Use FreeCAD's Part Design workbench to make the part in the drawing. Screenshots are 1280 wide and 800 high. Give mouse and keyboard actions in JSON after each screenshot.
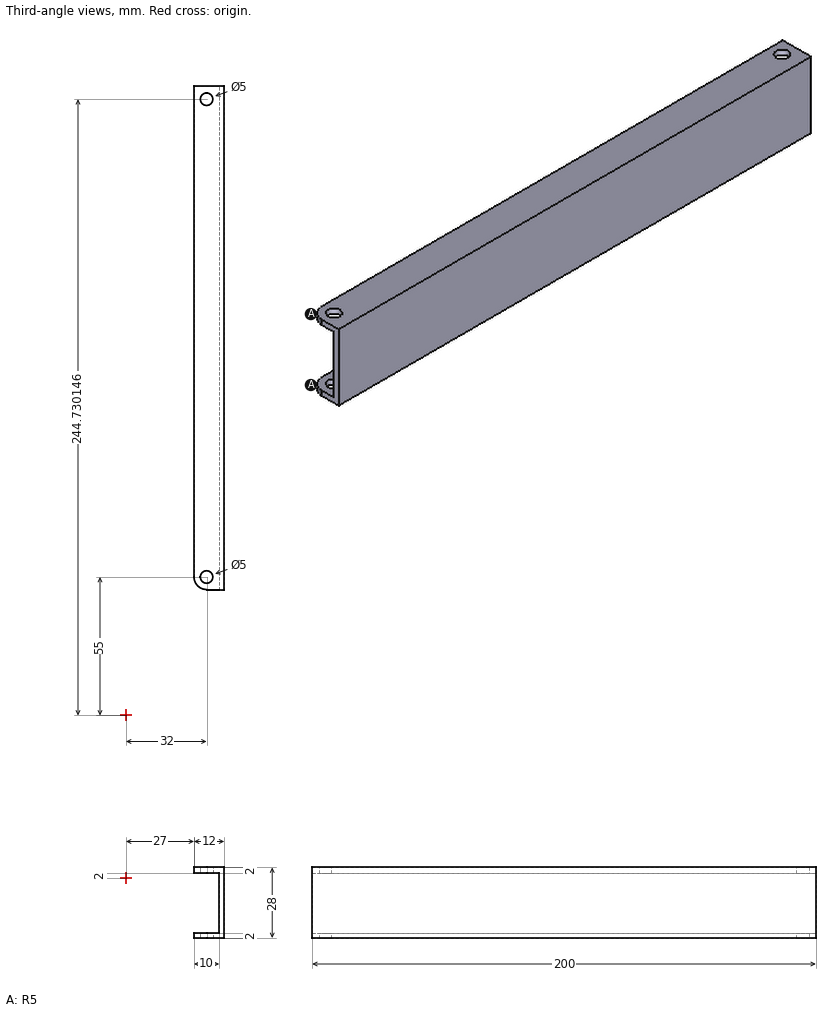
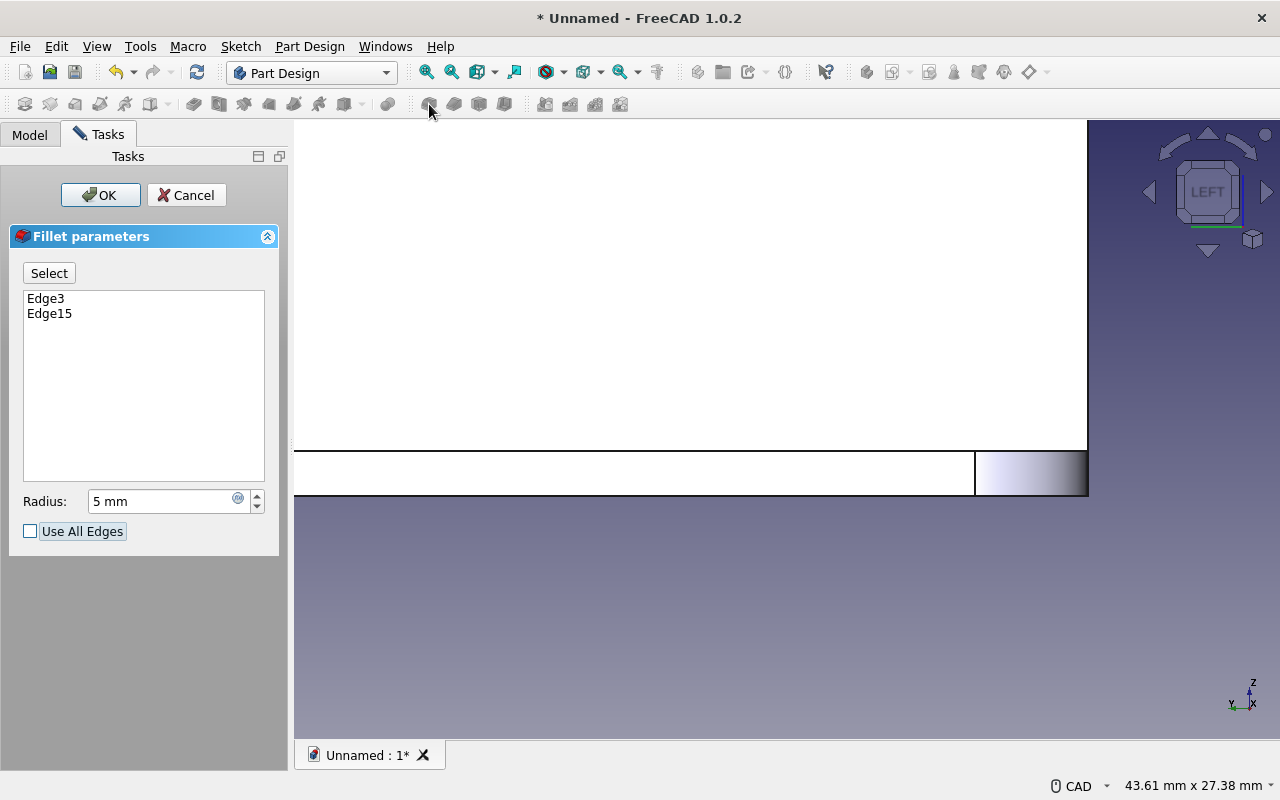
{"action": "left_click", "coordinate": [101, 195]}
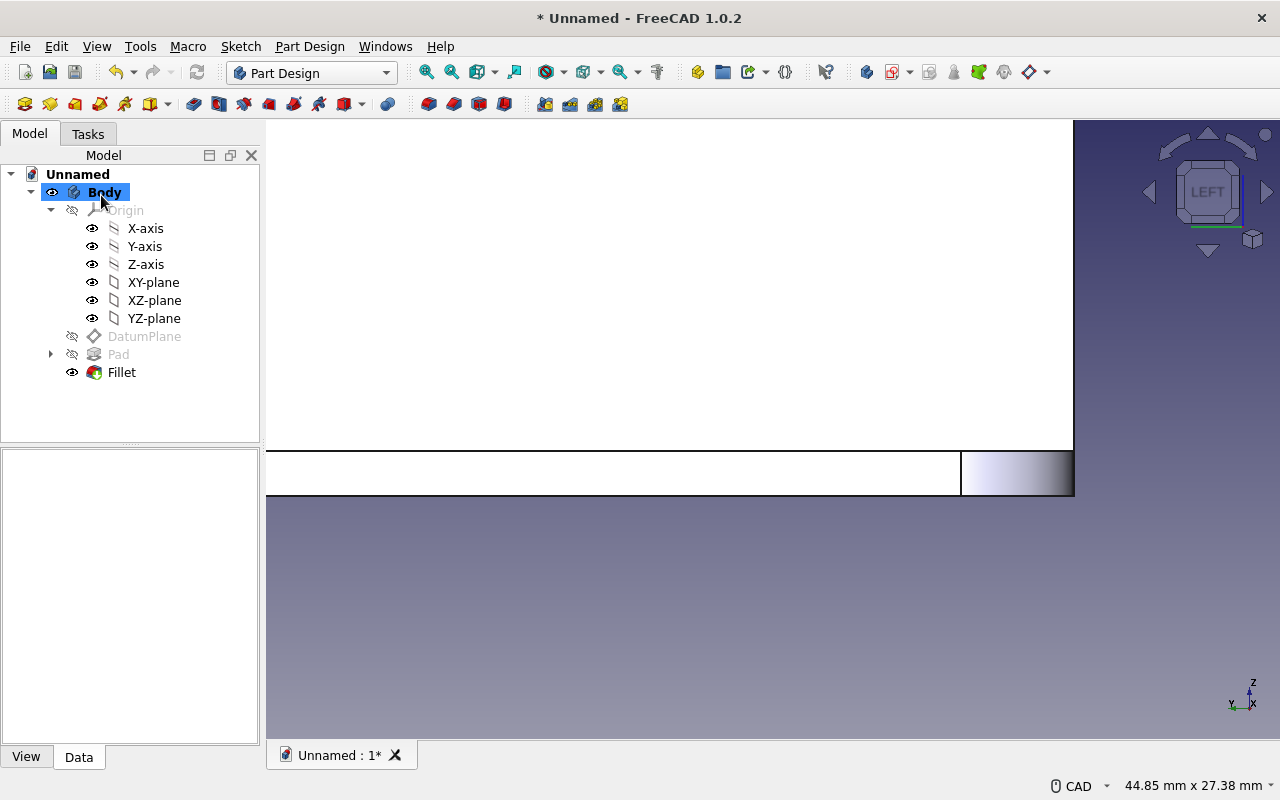
{"action": "left_click", "coordinate": [427, 72]}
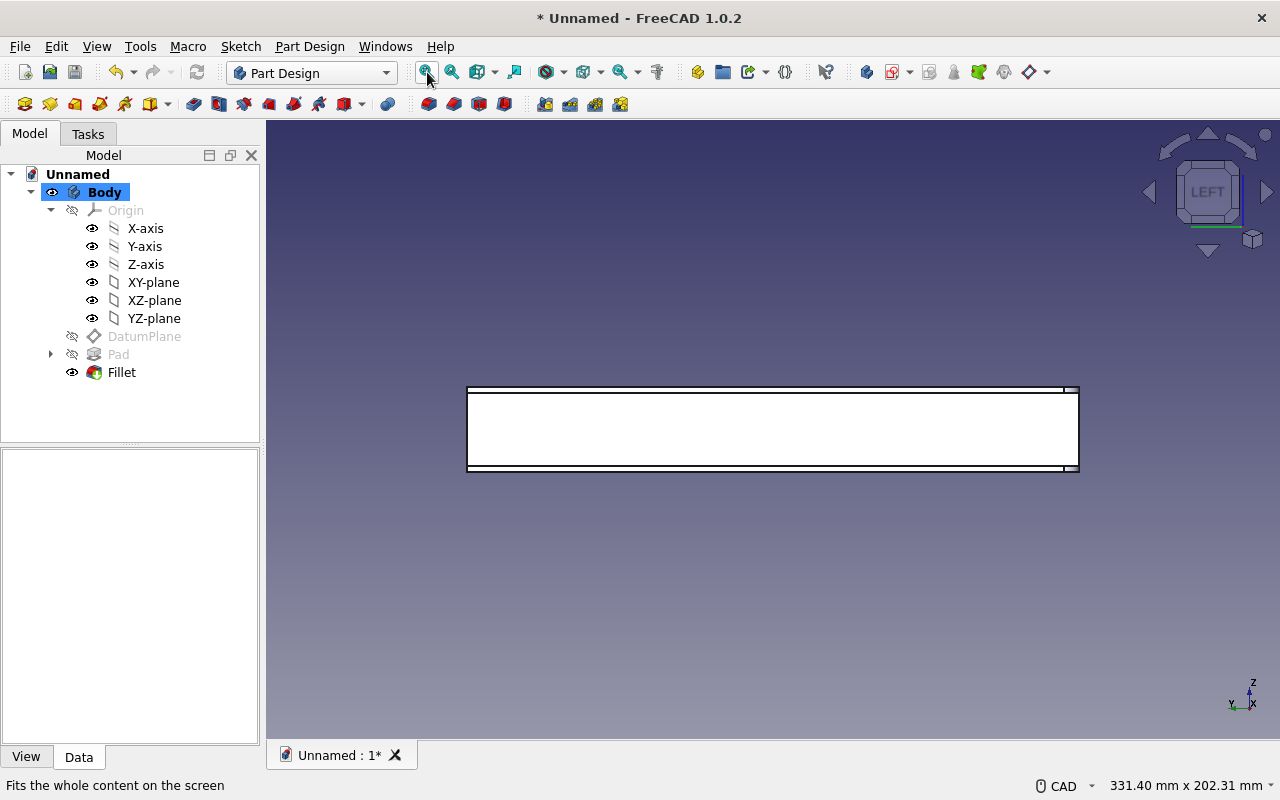
{"action": "left_click", "coordinate": [137, 282]}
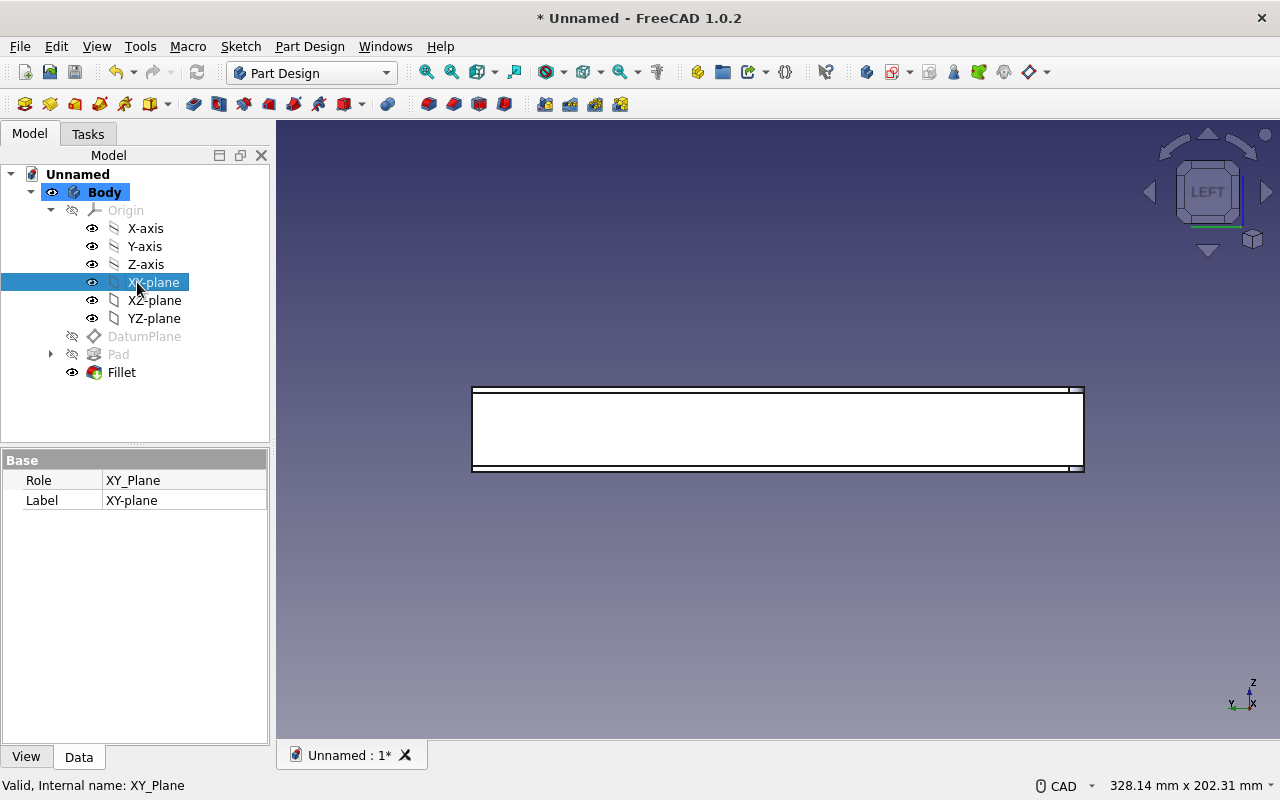
{"action": "left_click", "coordinate": [1028, 72]}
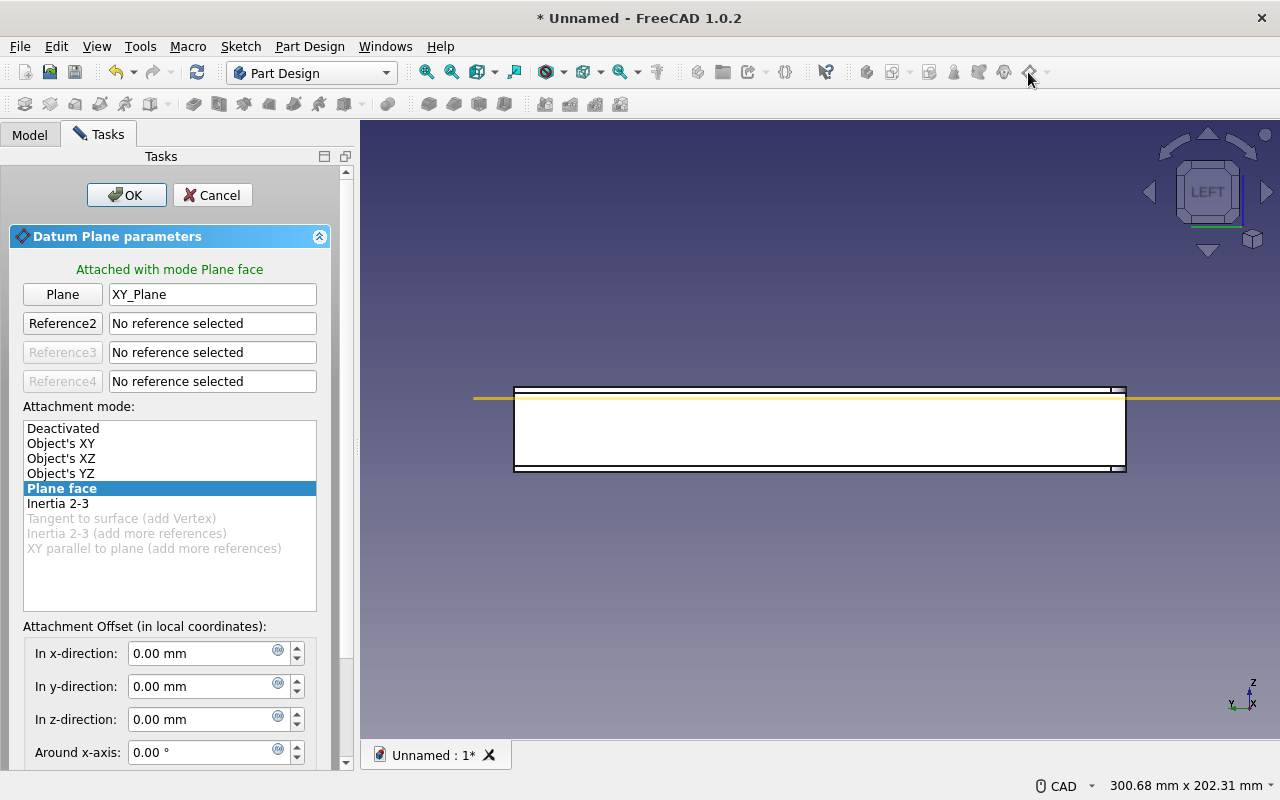
{"action": "triple_click", "coordinate": [210, 720]}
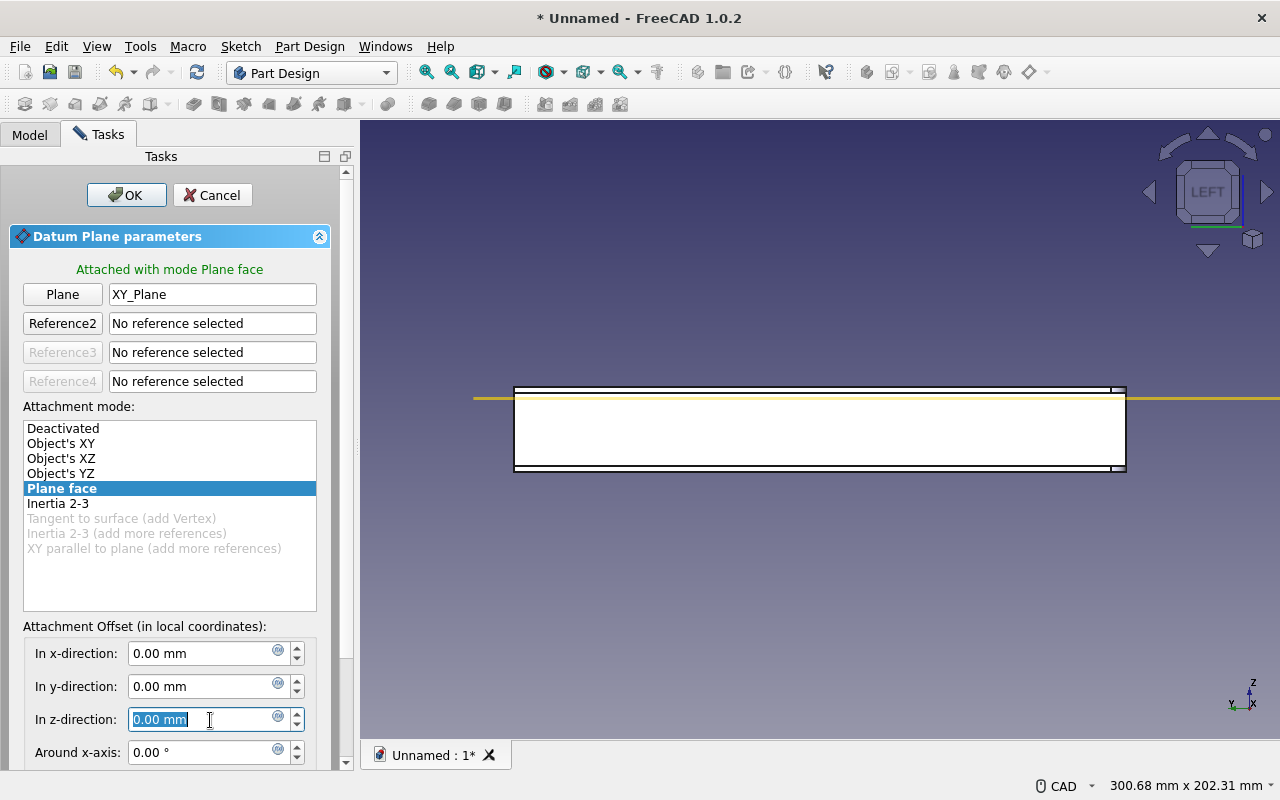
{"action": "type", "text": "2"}
{"action": "key", "text": "Tab"}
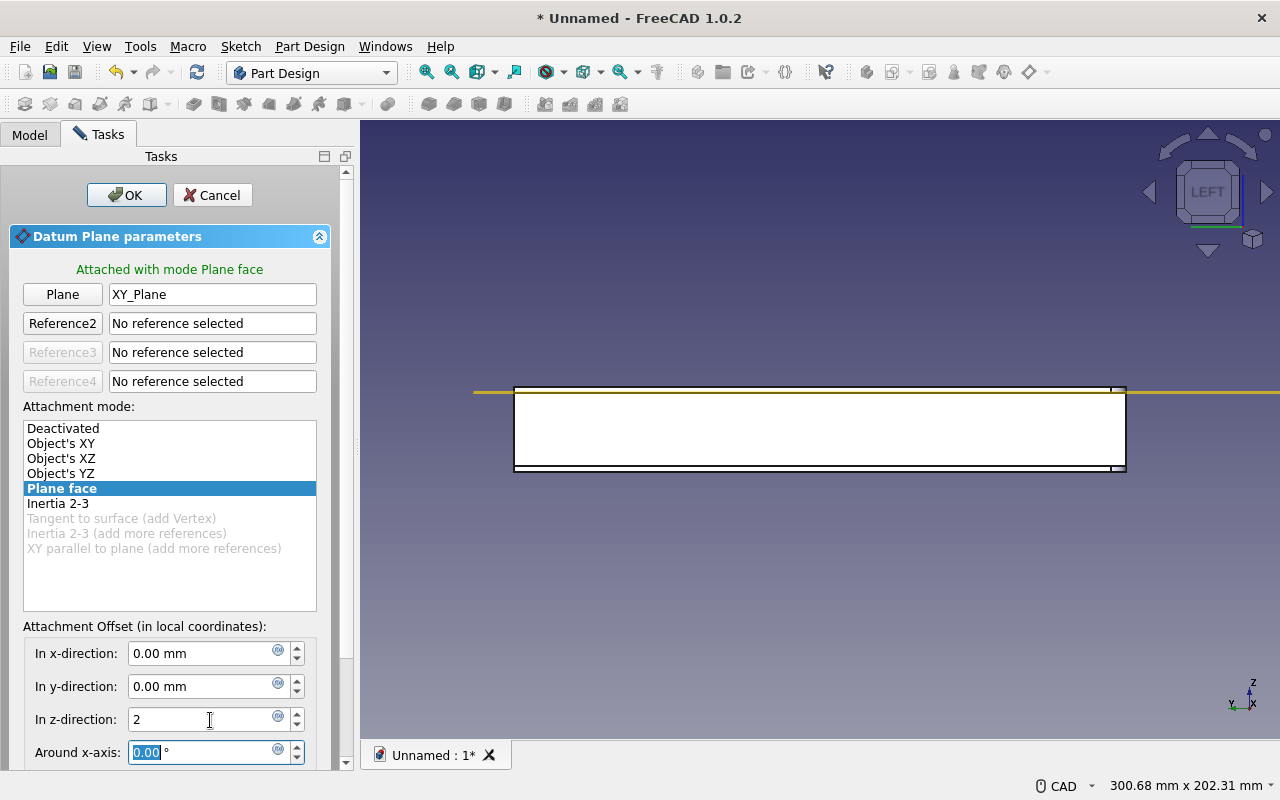
{"action": "left_click", "coordinate": [127, 195]}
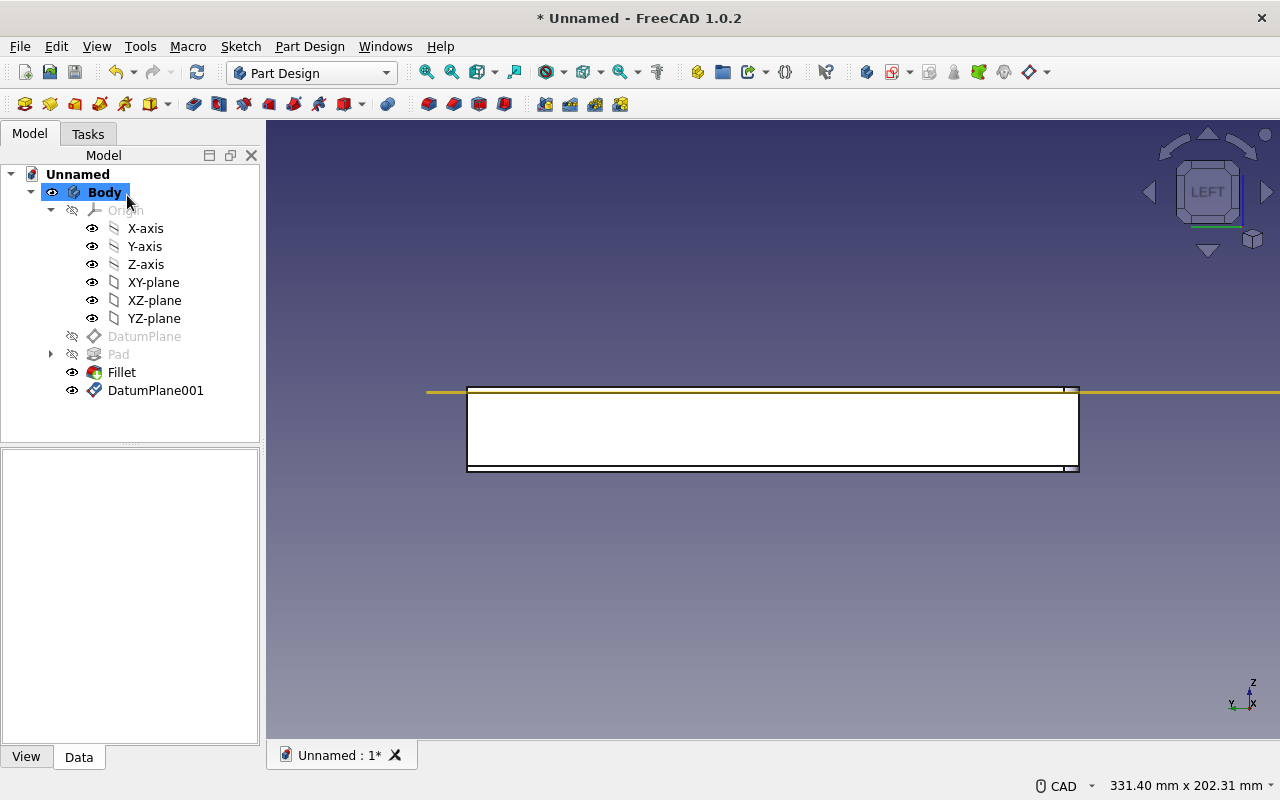
{"action": "left_click", "coordinate": [117, 390]}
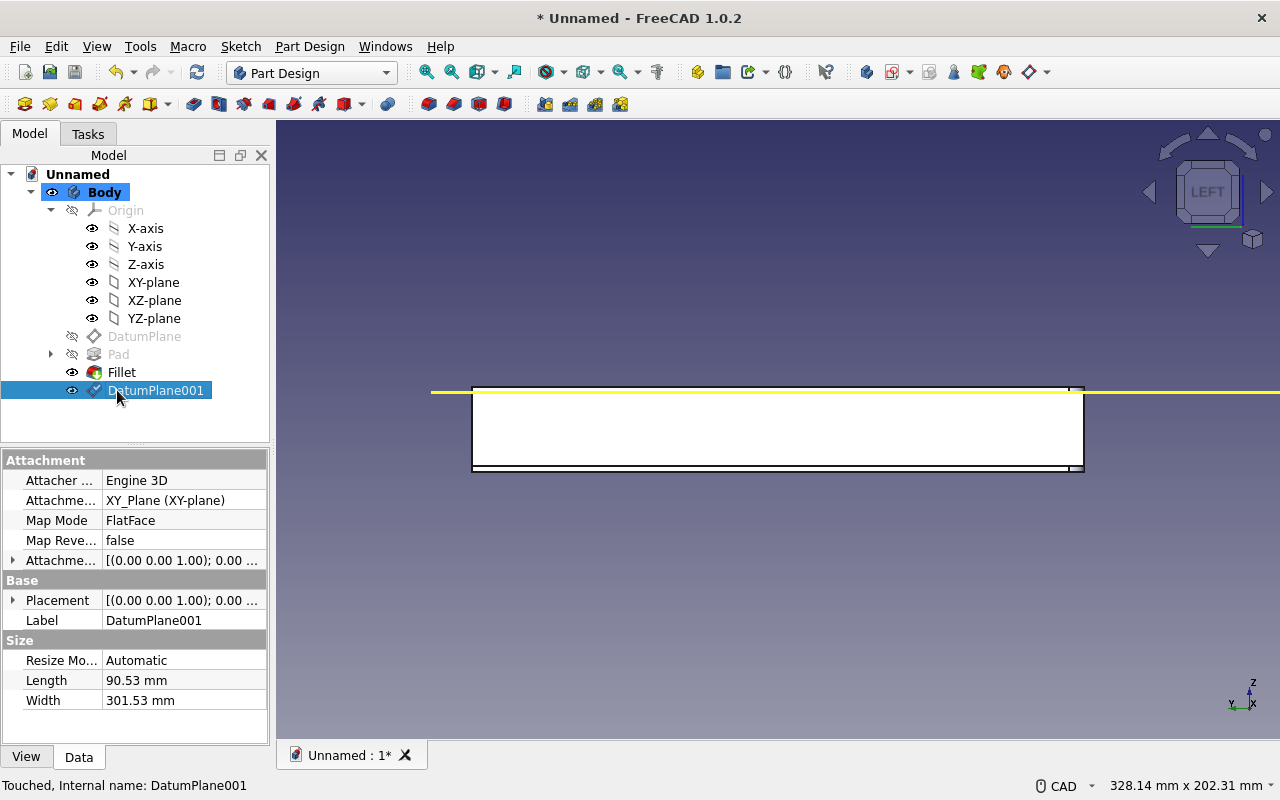
{"action": "left_click", "coordinate": [892, 72]}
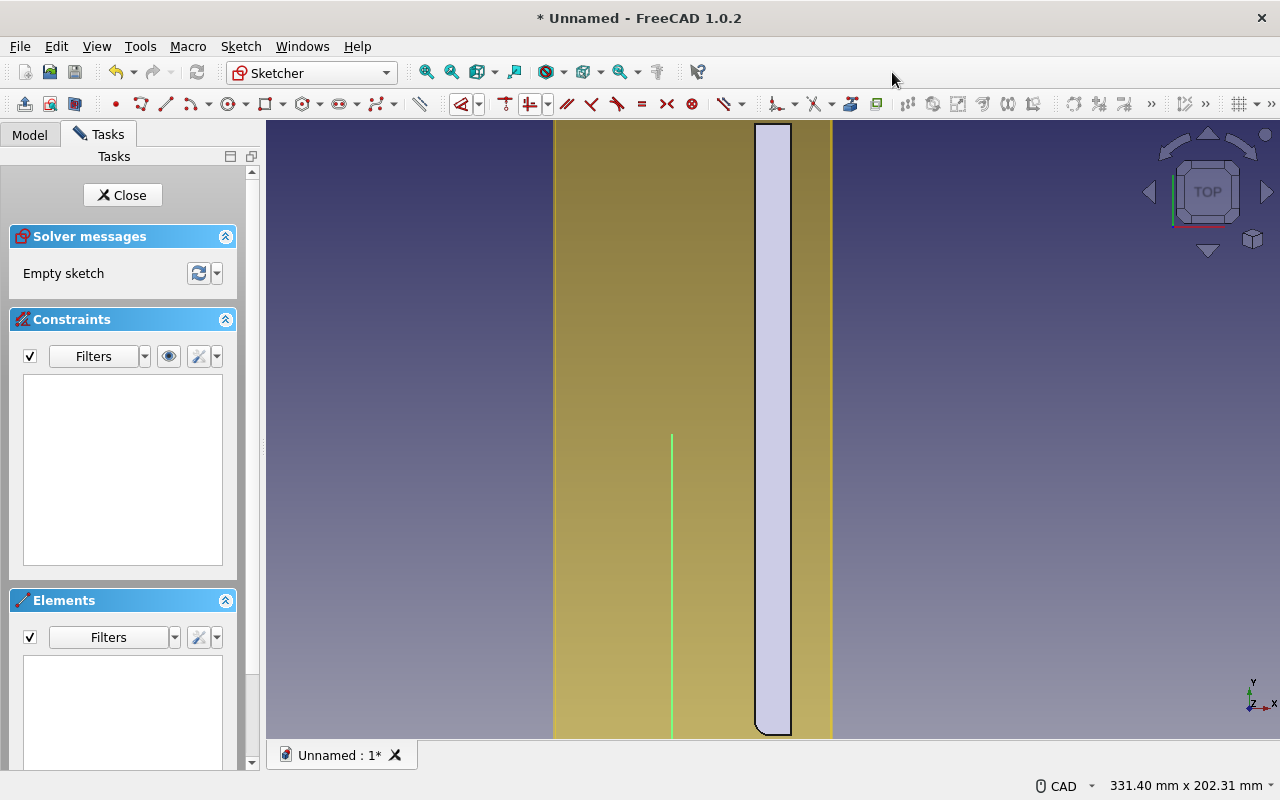
{"action": "left_click", "coordinate": [75, 104]}